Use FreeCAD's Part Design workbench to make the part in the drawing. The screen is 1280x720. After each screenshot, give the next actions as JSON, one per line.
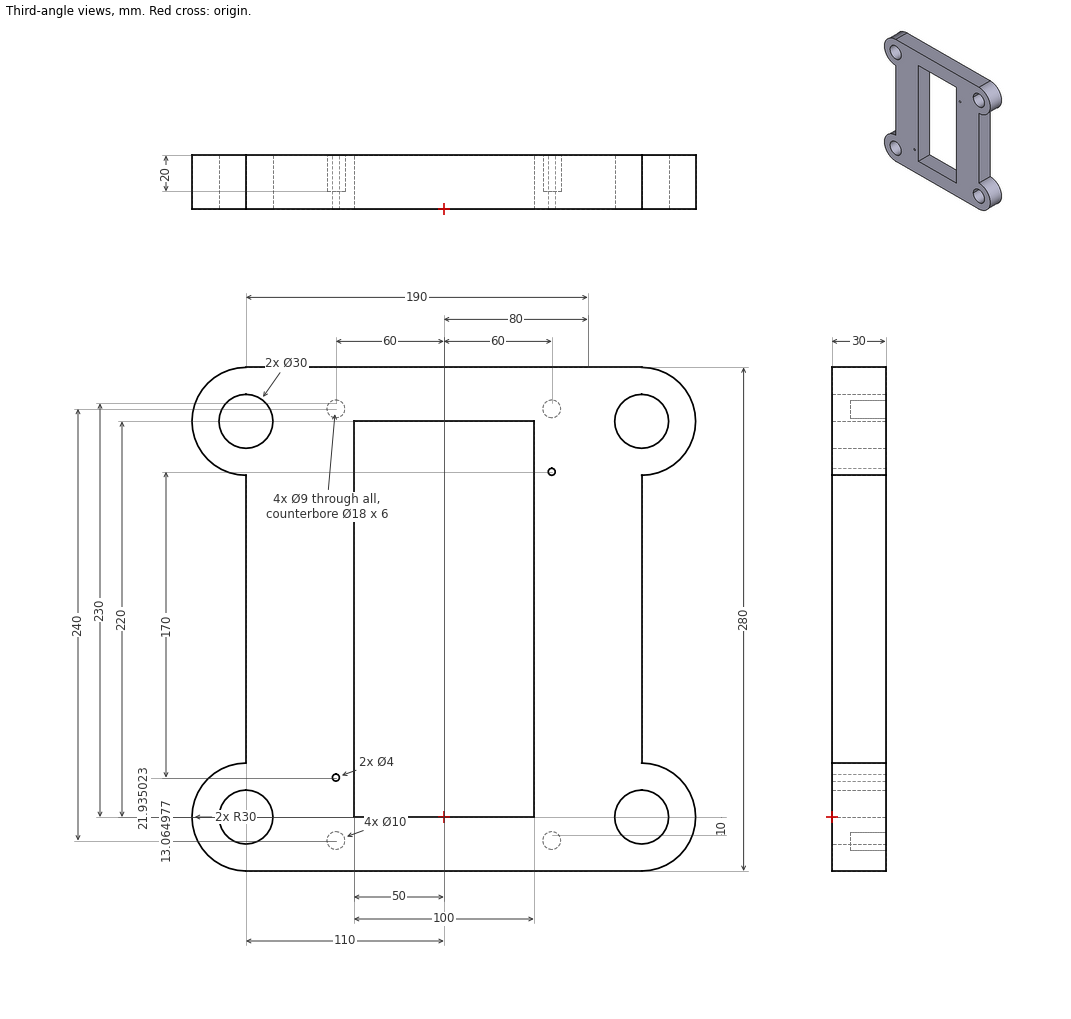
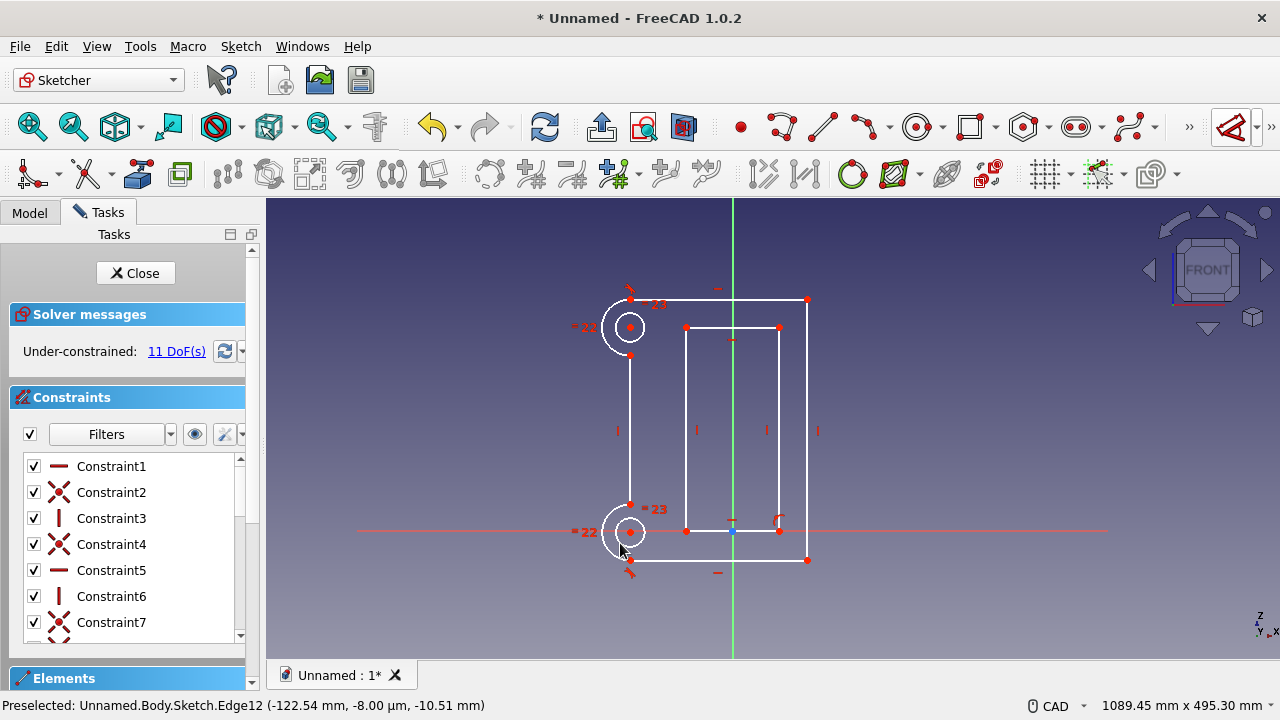
{"action": "left_click", "coordinate": [630, 533]}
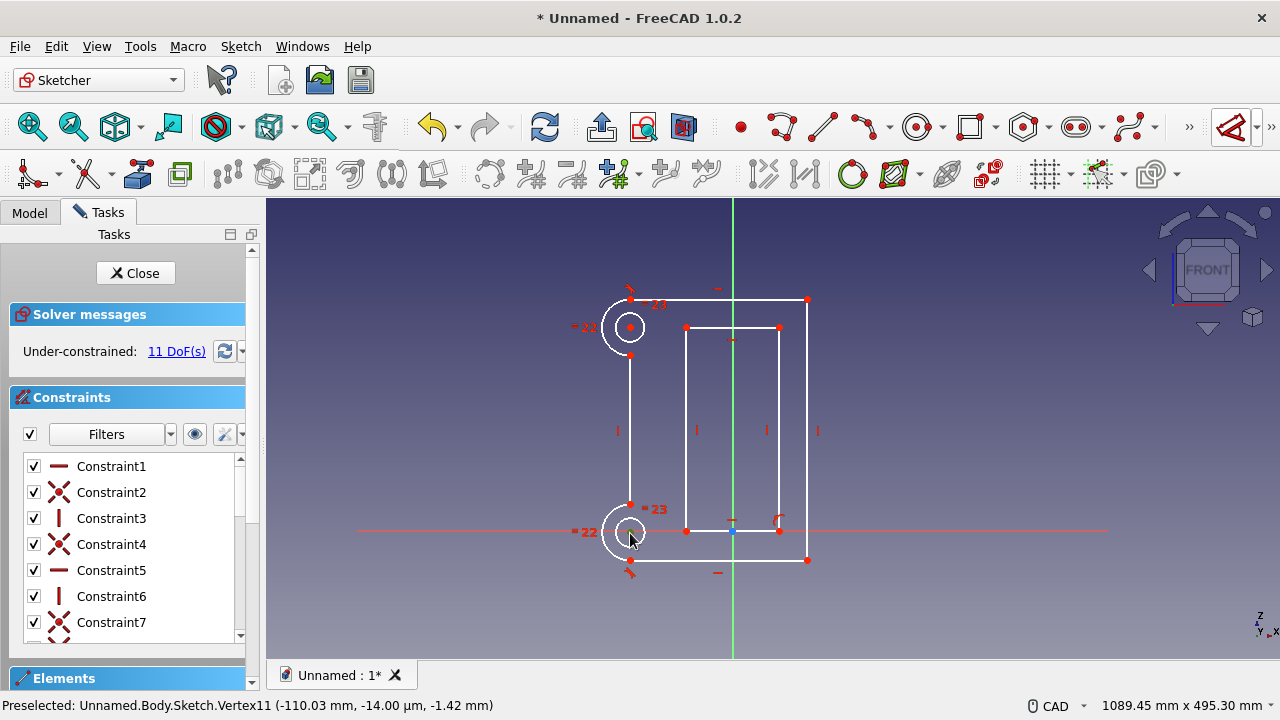
{"action": "left_click", "coordinate": [353, 531]}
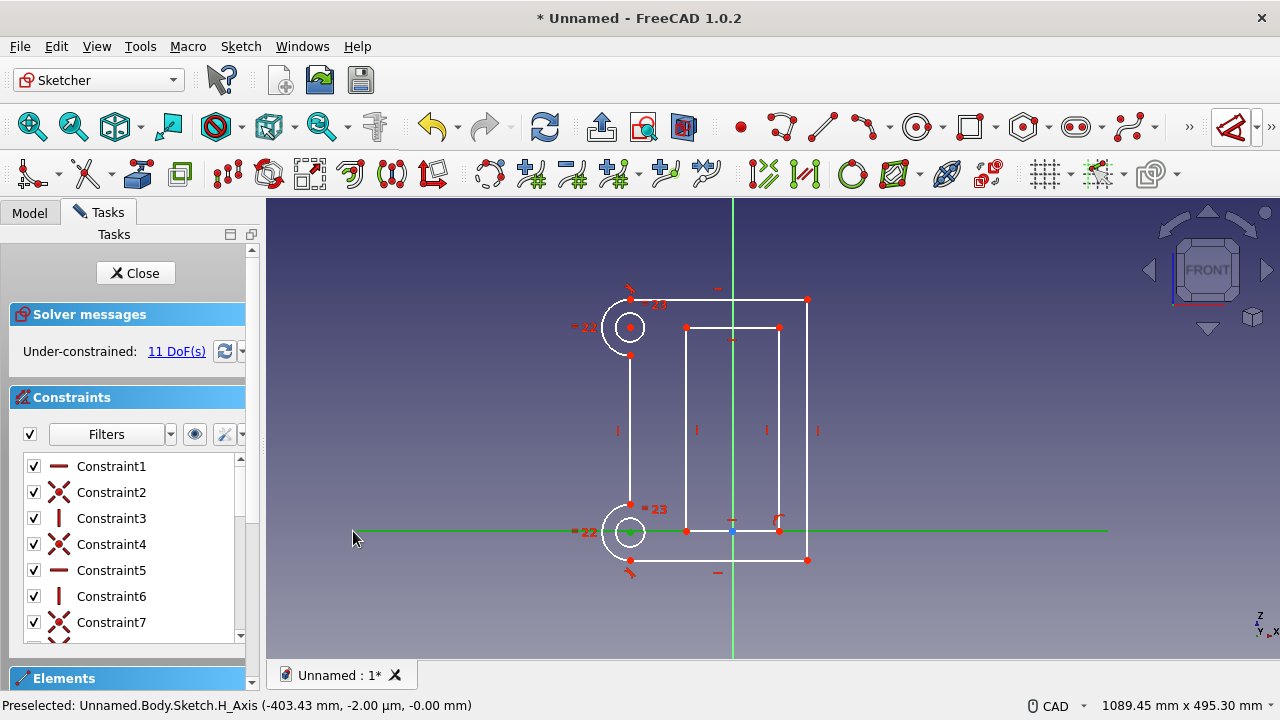
{"action": "key", "text": "c"}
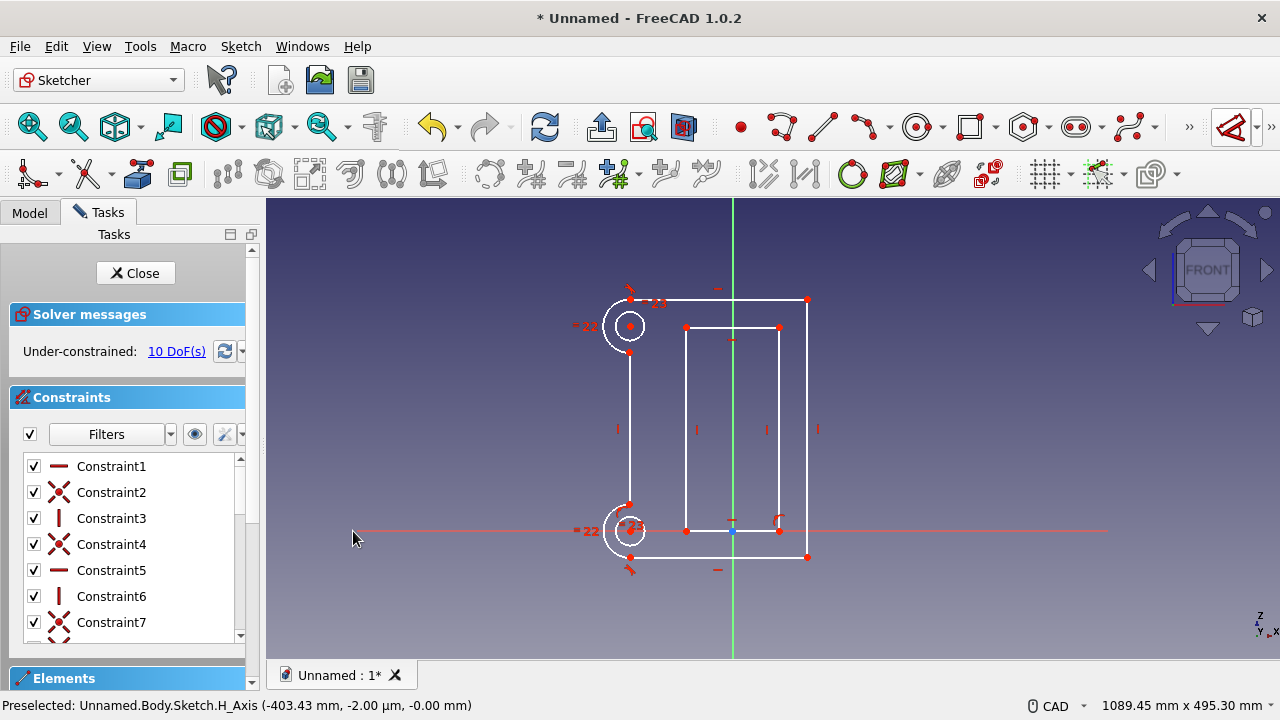
{"action": "key", "text": "d"}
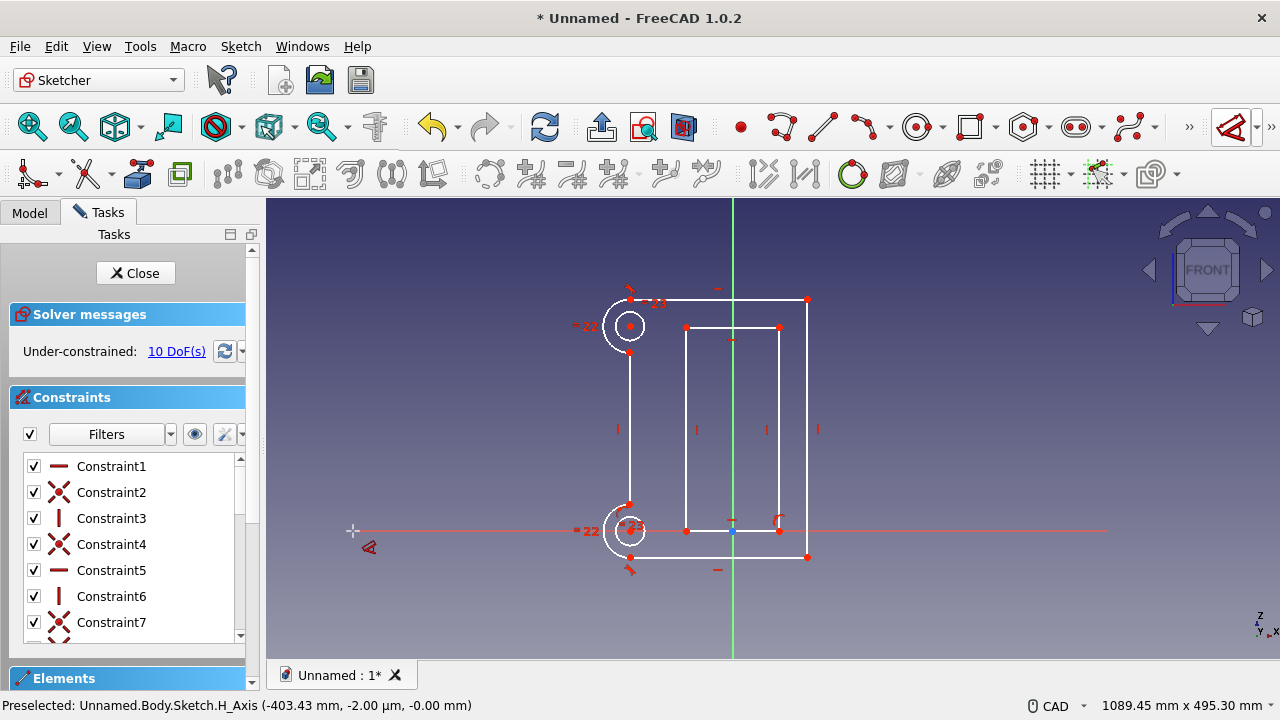
{"action": "scroll", "coordinate": [609, 516], "scroll_direction": "up", "scroll_amount": 2}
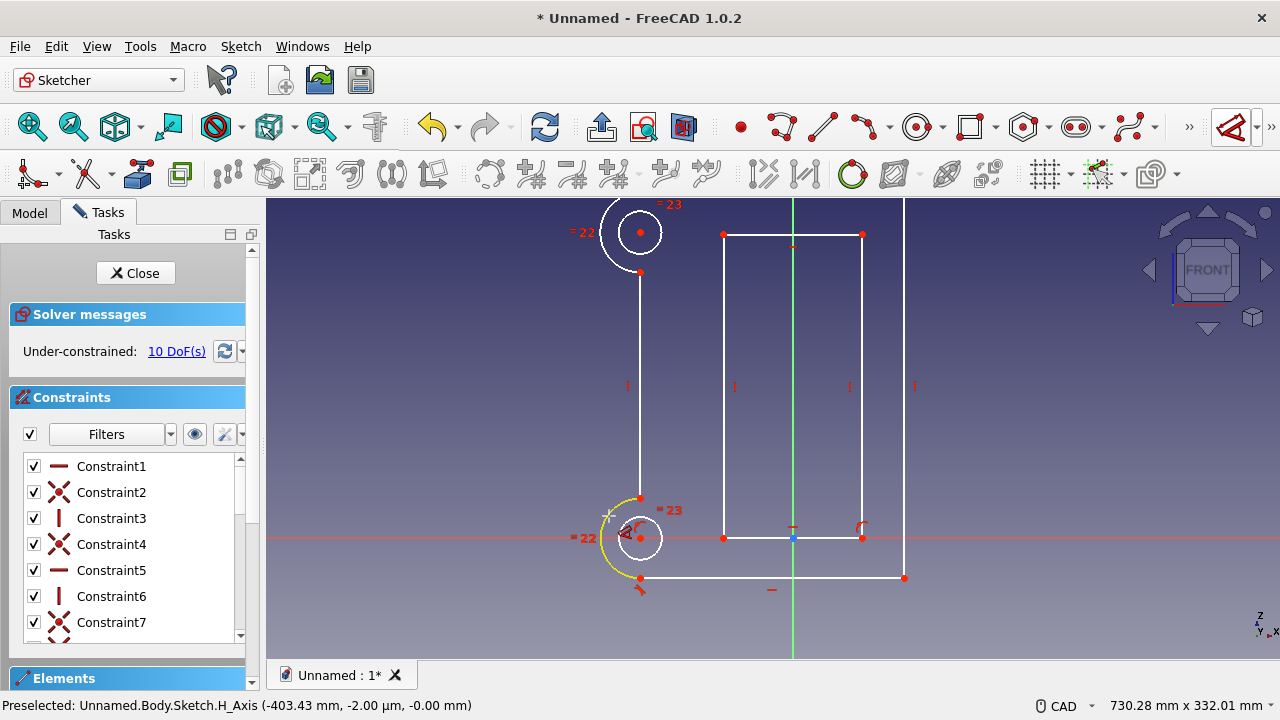
{"action": "left_click", "coordinate": [608, 515]}
{"action": "left_click", "coordinate": [582, 496]}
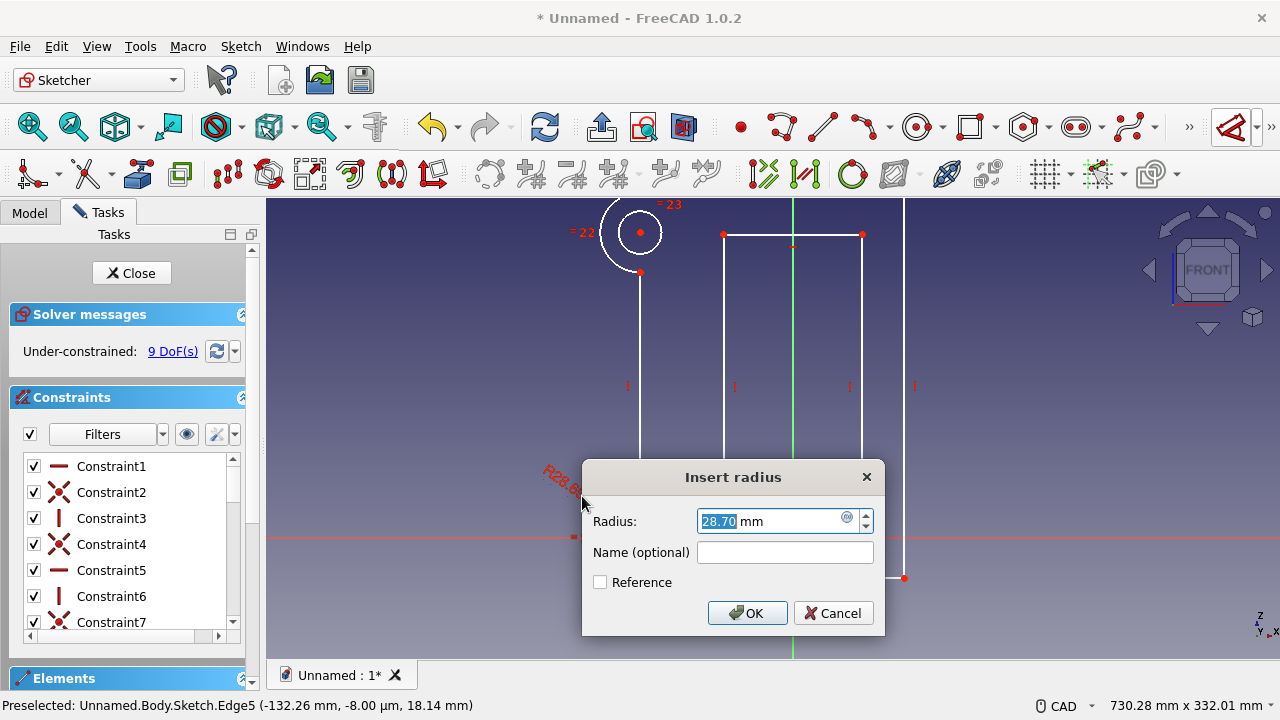
{"action": "type", "text": "30"}
{"action": "key", "text": "Return"}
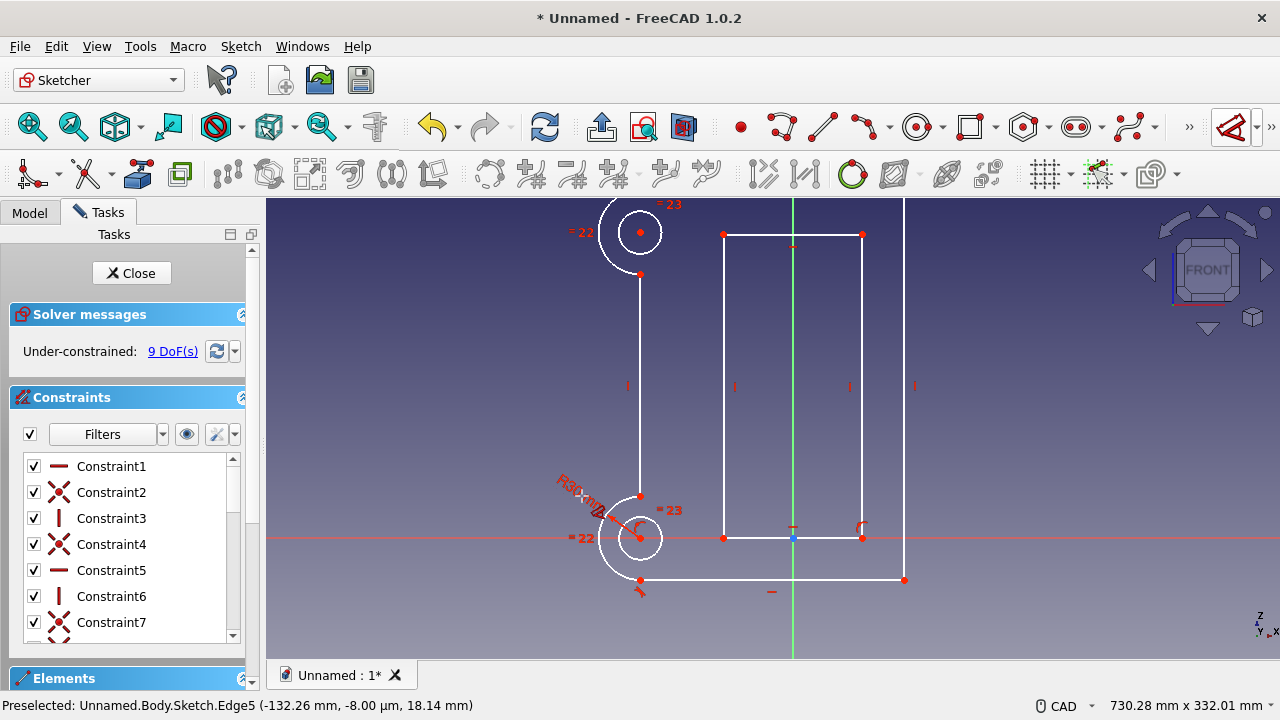
{"action": "left_click", "coordinate": [625, 248]}
{"action": "left_click", "coordinate": [678, 270]}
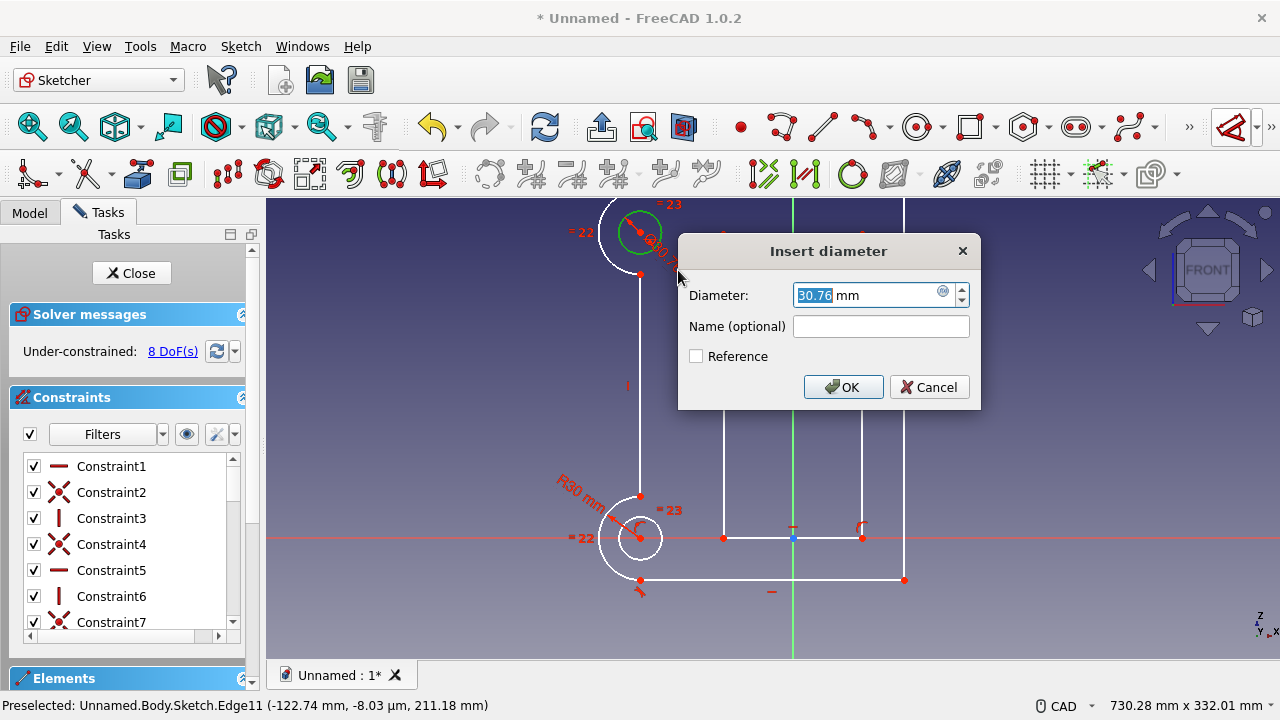
{"action": "type", "text": "30"}
{"action": "key", "text": "Return"}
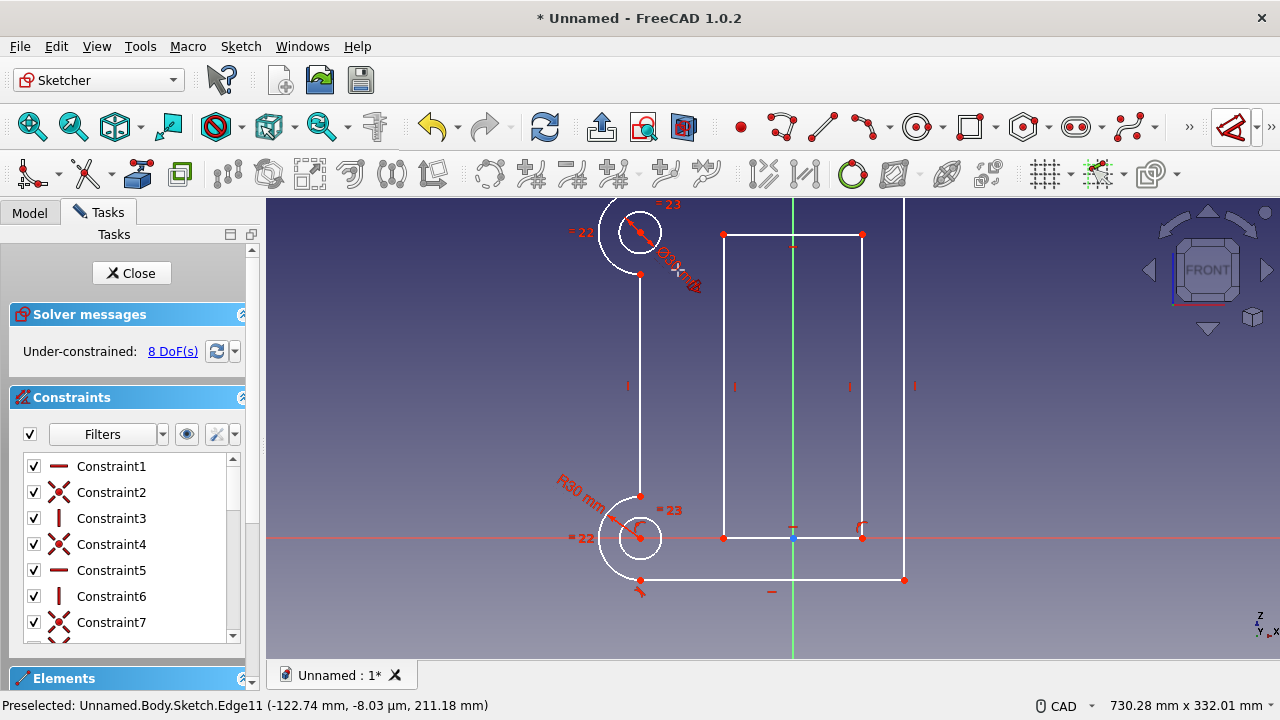
{"action": "scroll", "coordinate": [609, 516], "scroll_direction": "down", "scroll_amount": 2}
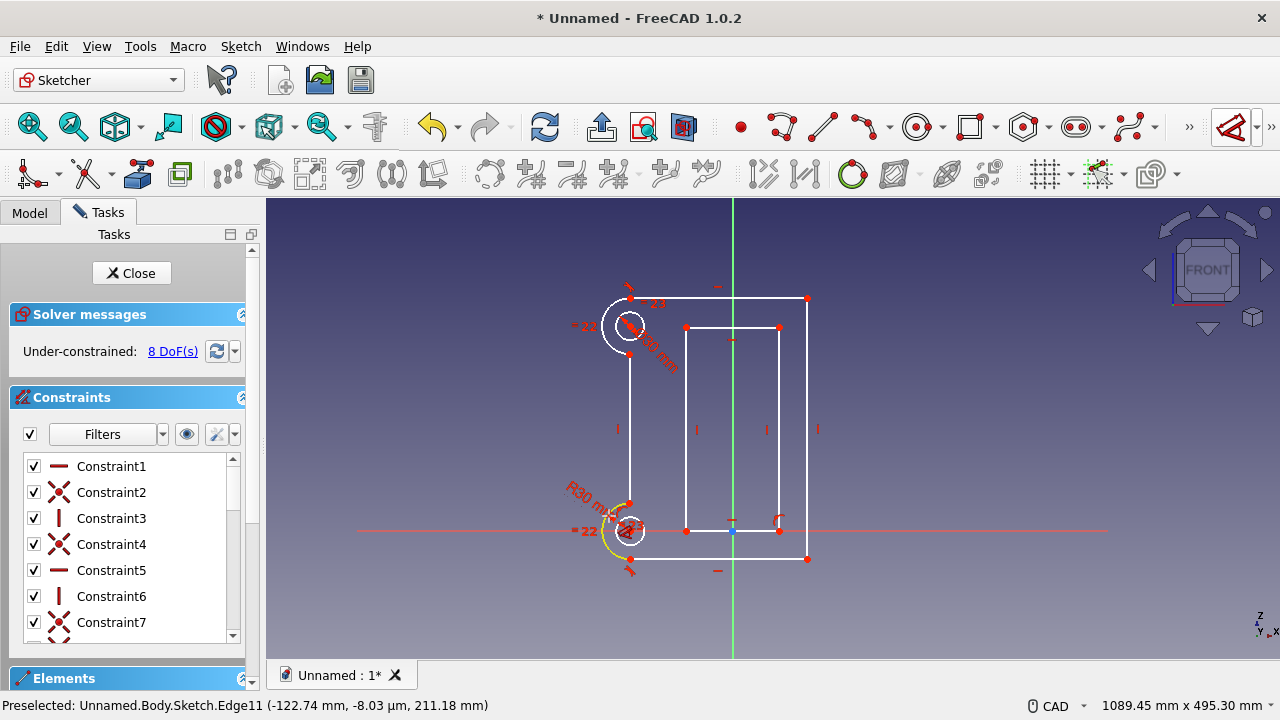
{"action": "left_click", "coordinate": [683, 298]}
{"action": "left_click", "coordinate": [719, 264]}